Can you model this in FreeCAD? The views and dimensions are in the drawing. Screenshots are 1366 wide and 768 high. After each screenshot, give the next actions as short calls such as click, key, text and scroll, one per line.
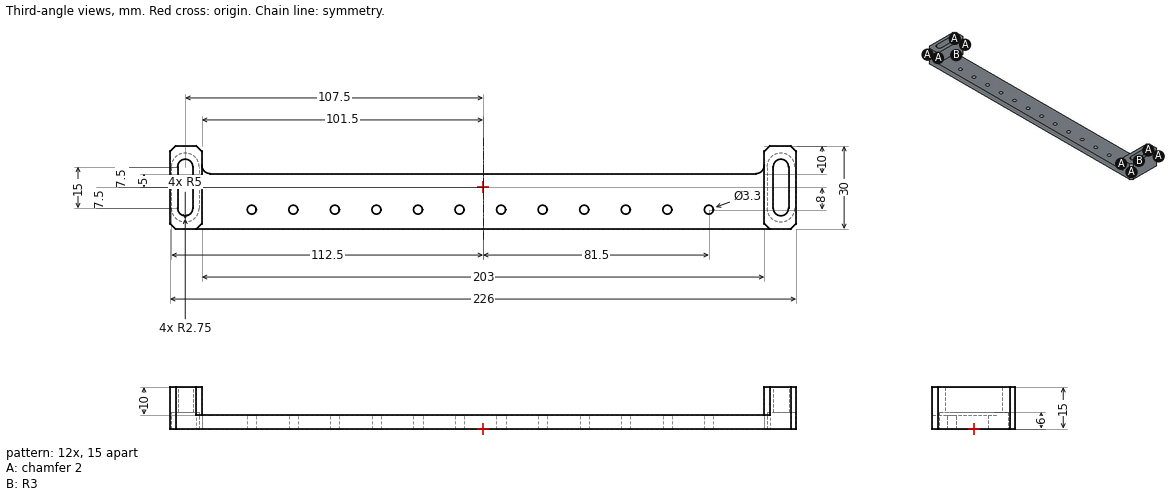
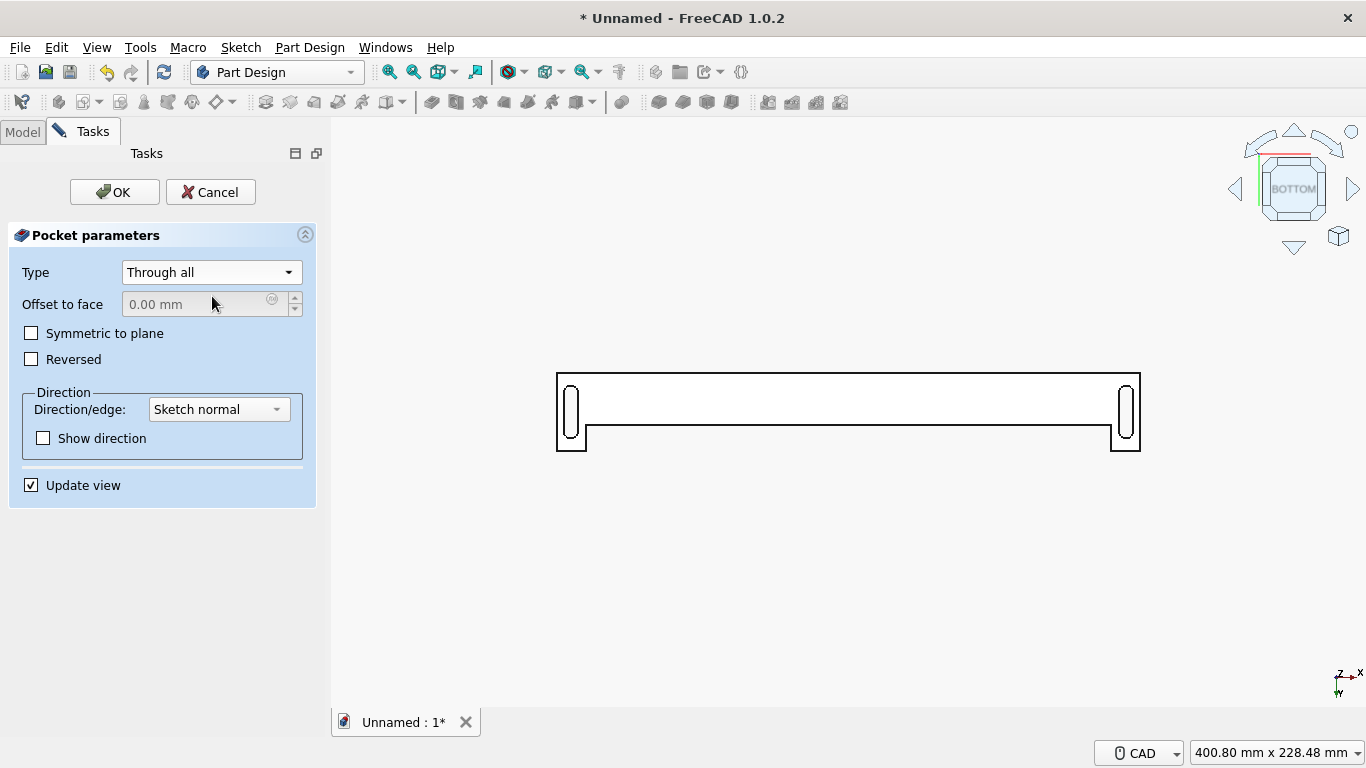
click(115, 192)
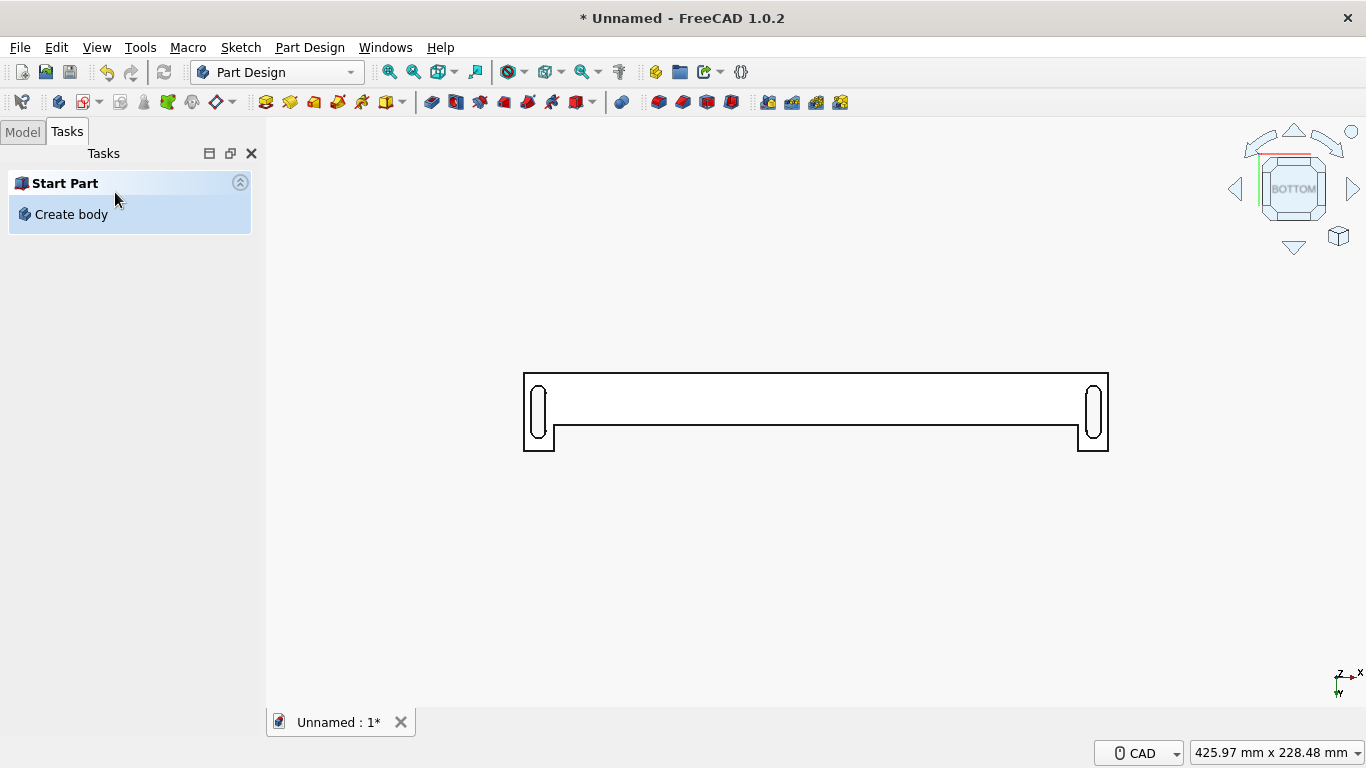
click(84, 102)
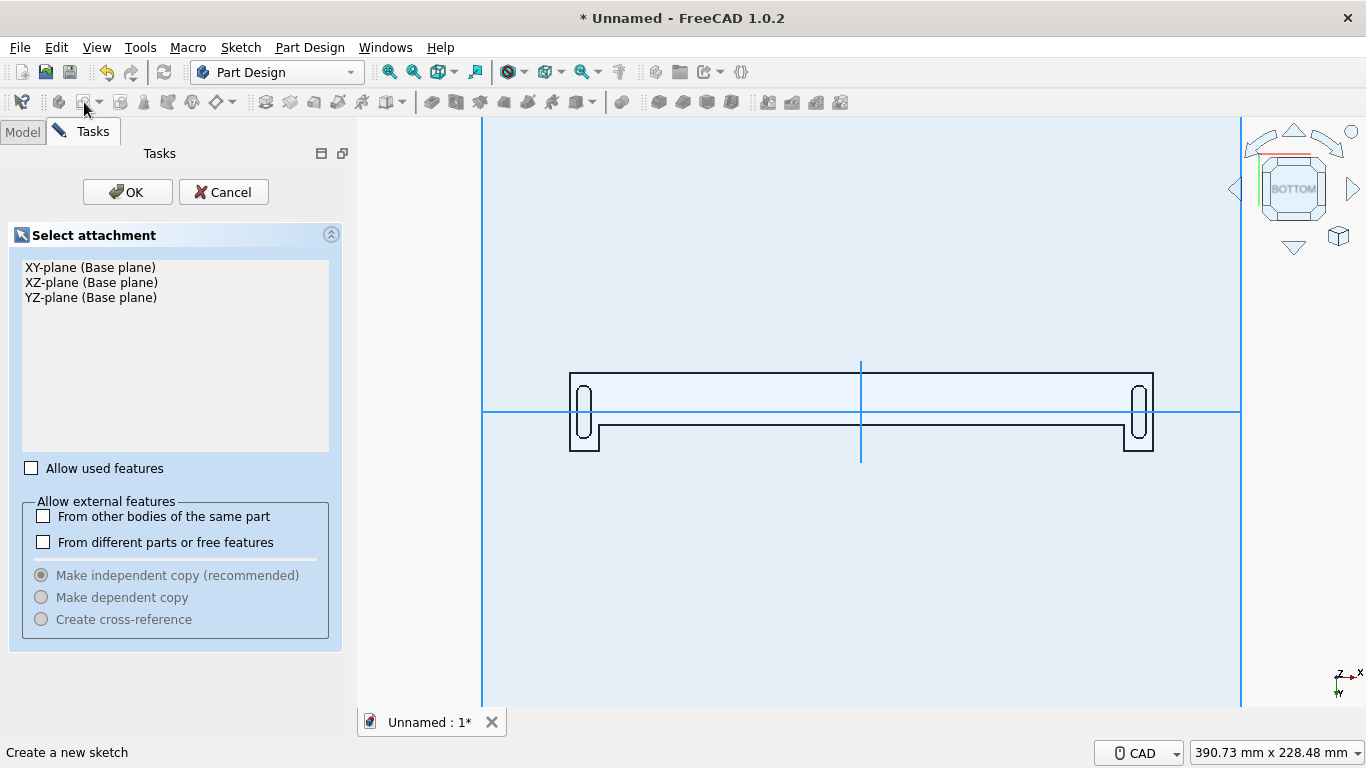
click(82, 268)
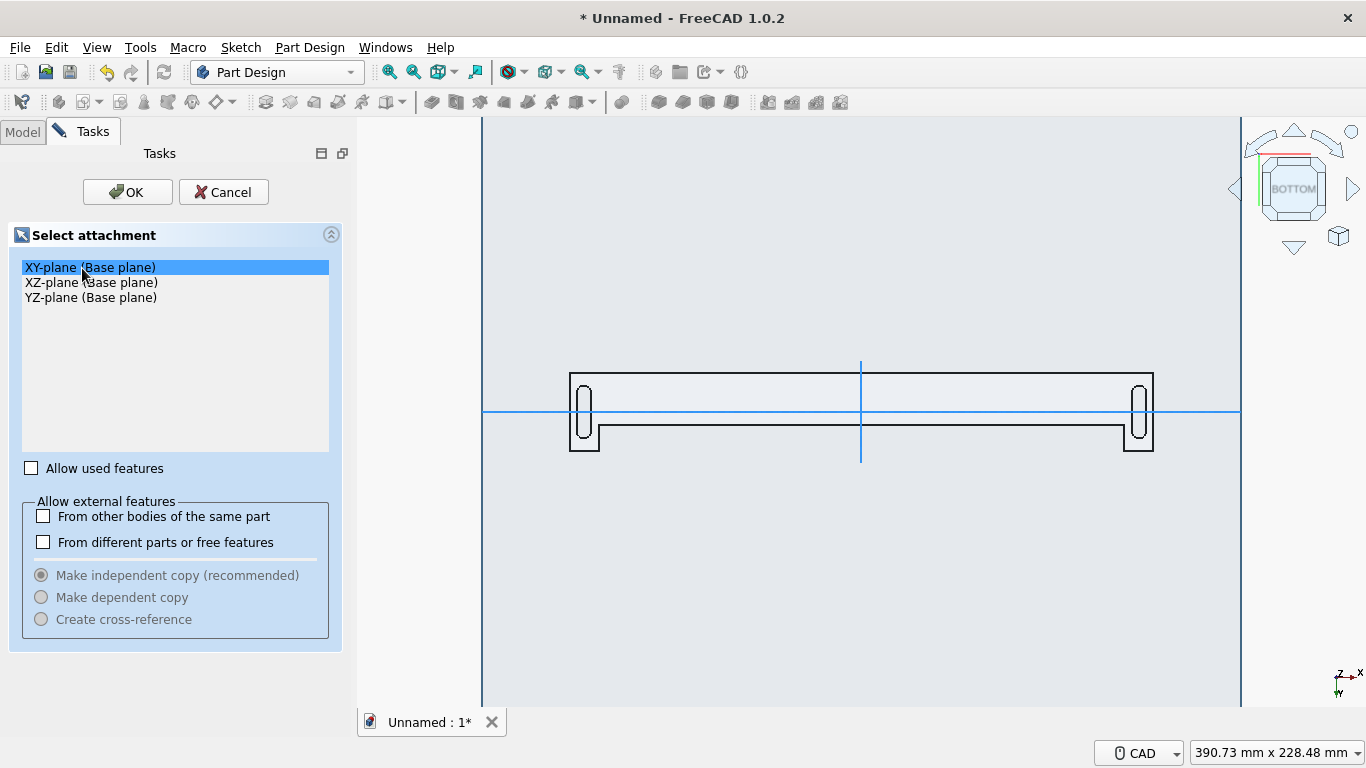
click(128, 192)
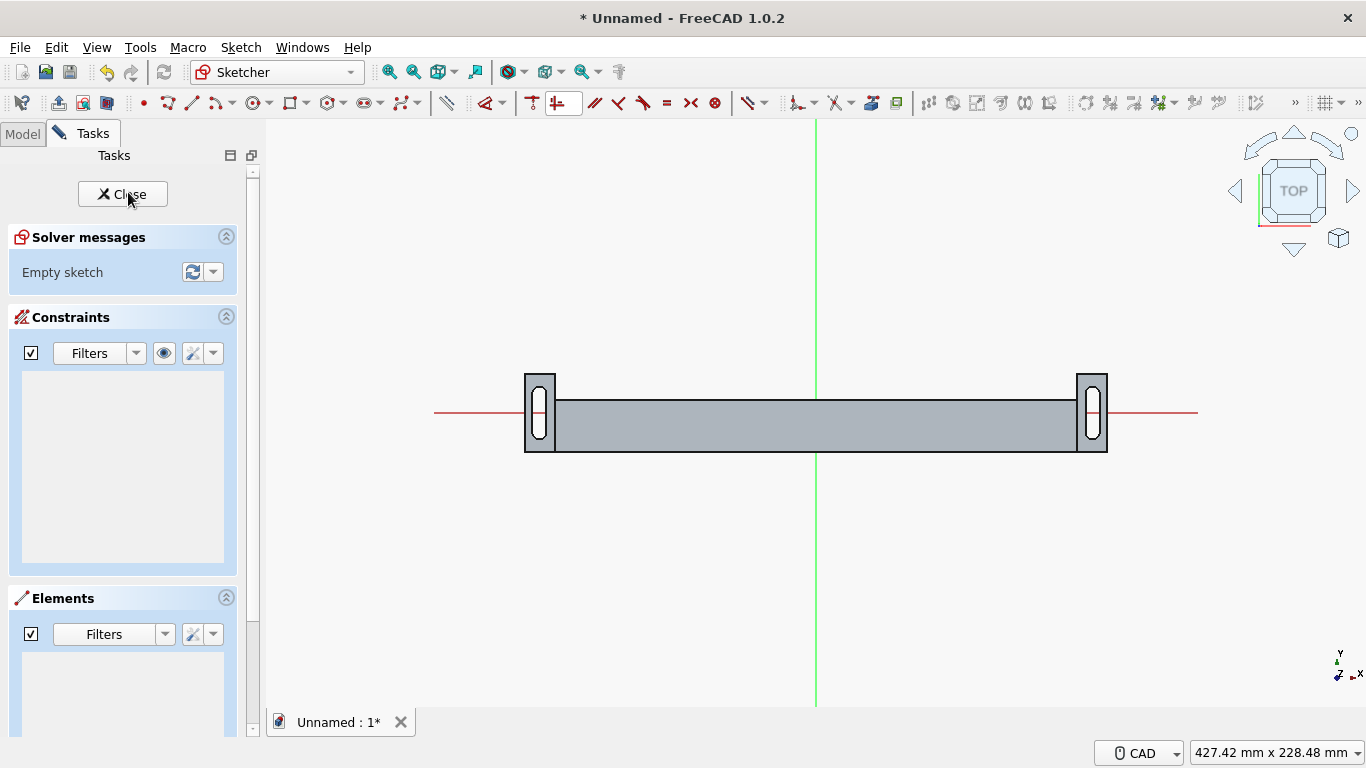
key(q)
key(s)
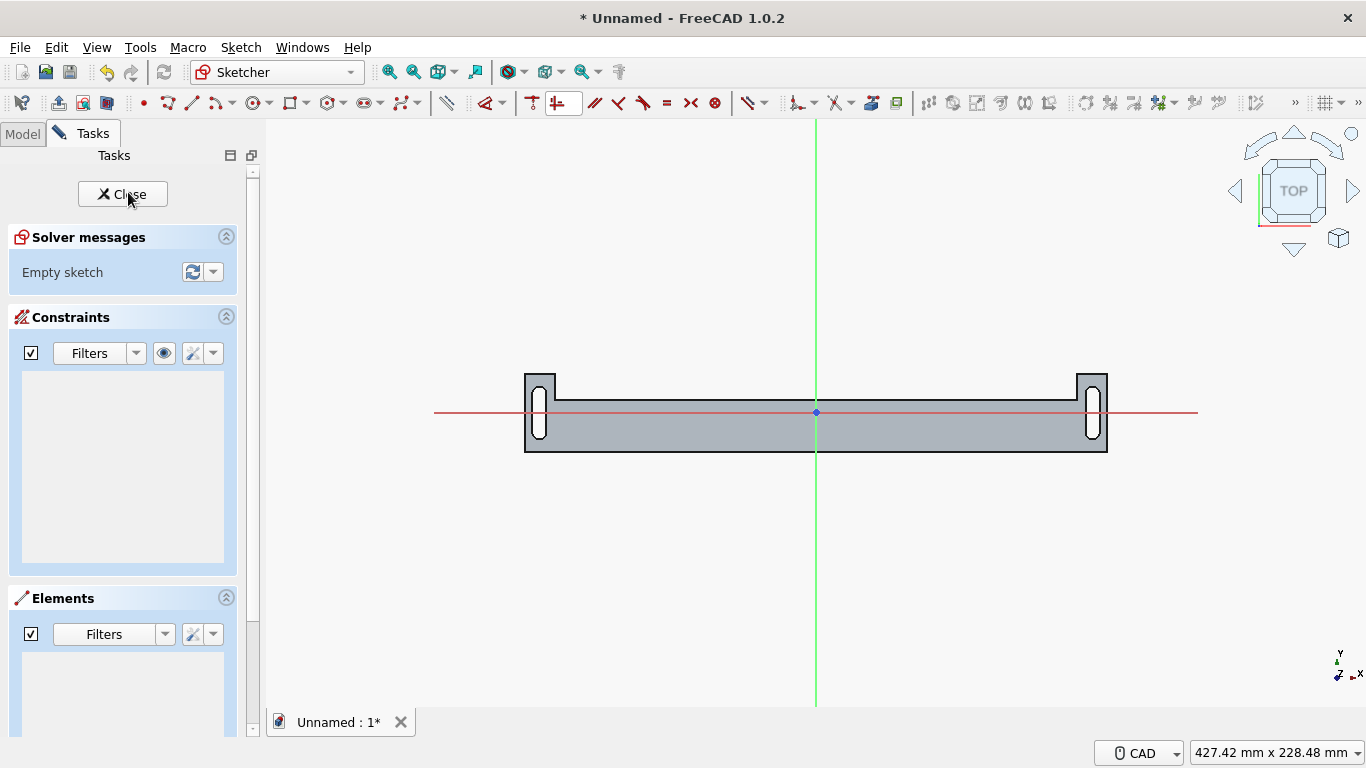
key(g)
key(s)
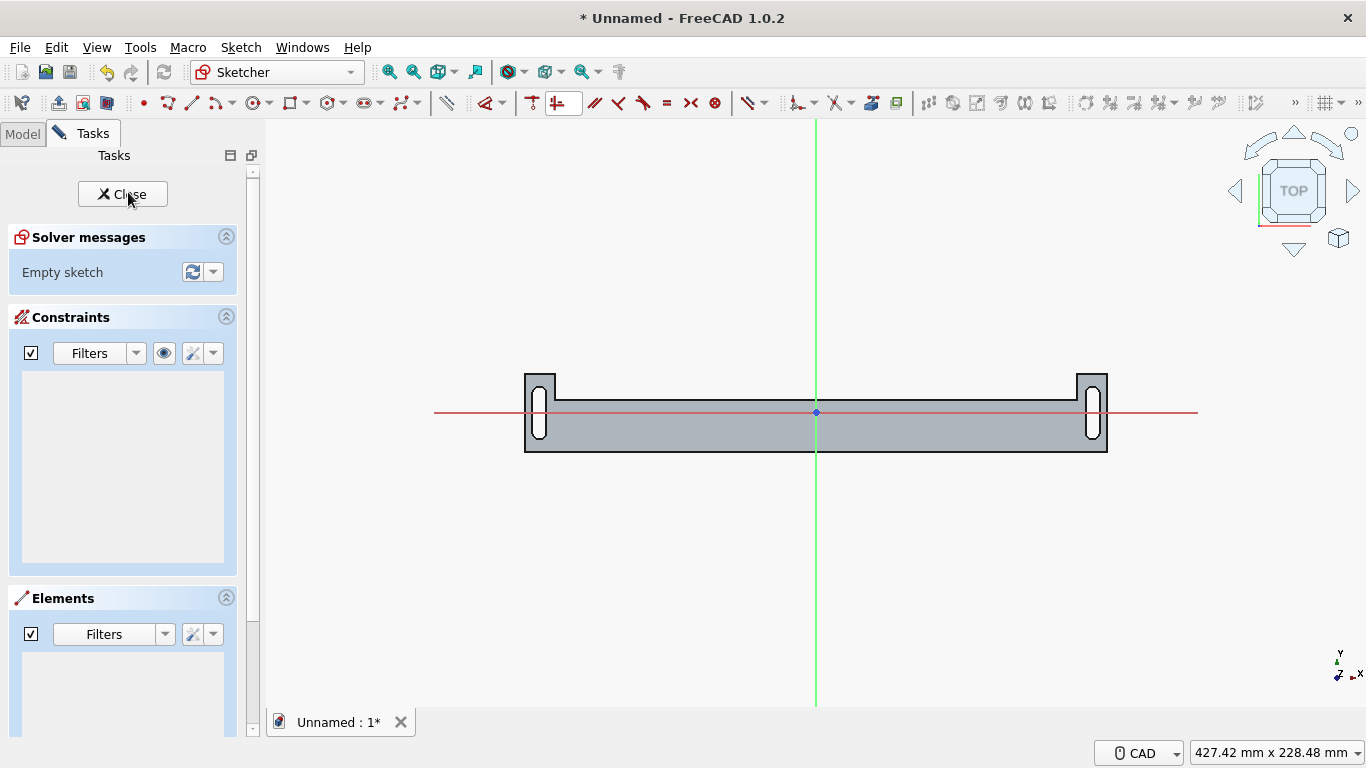
scroll(539, 432, up, 3)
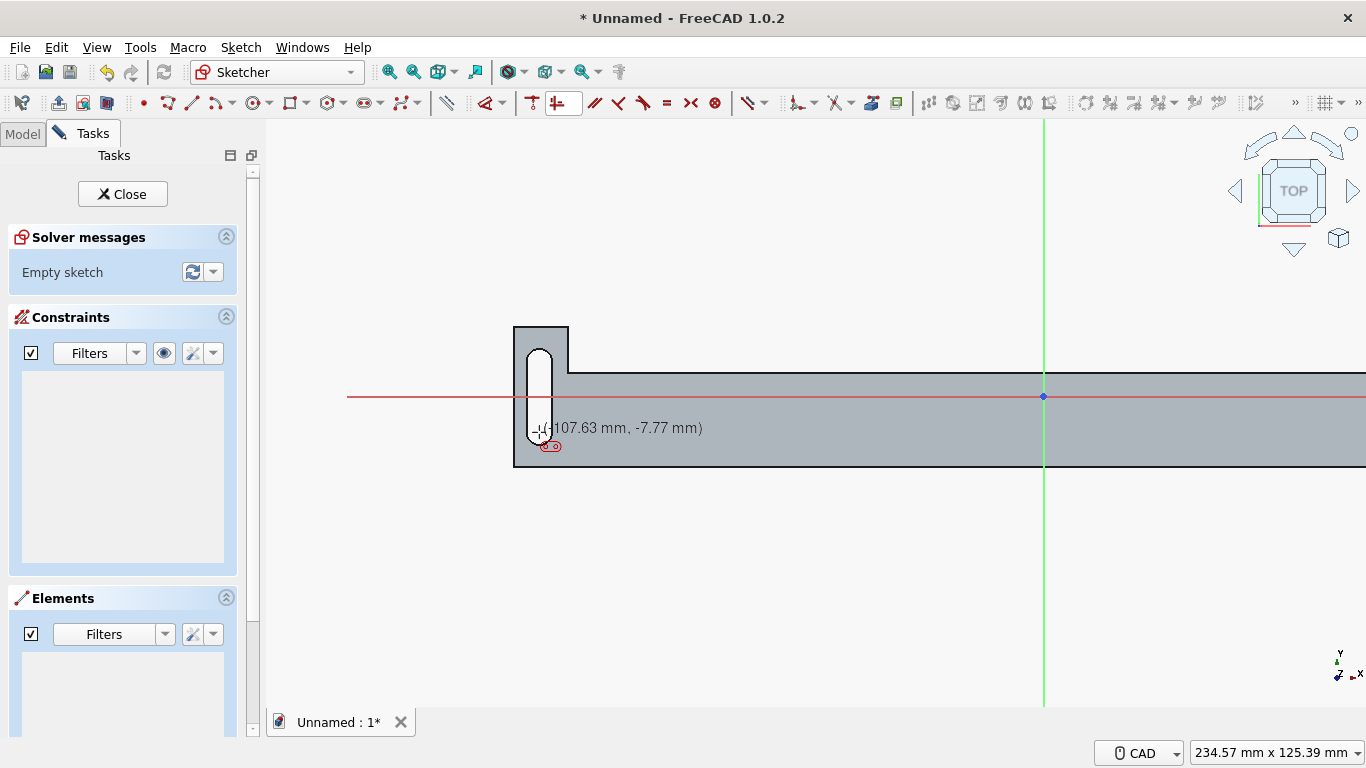
click(539, 432)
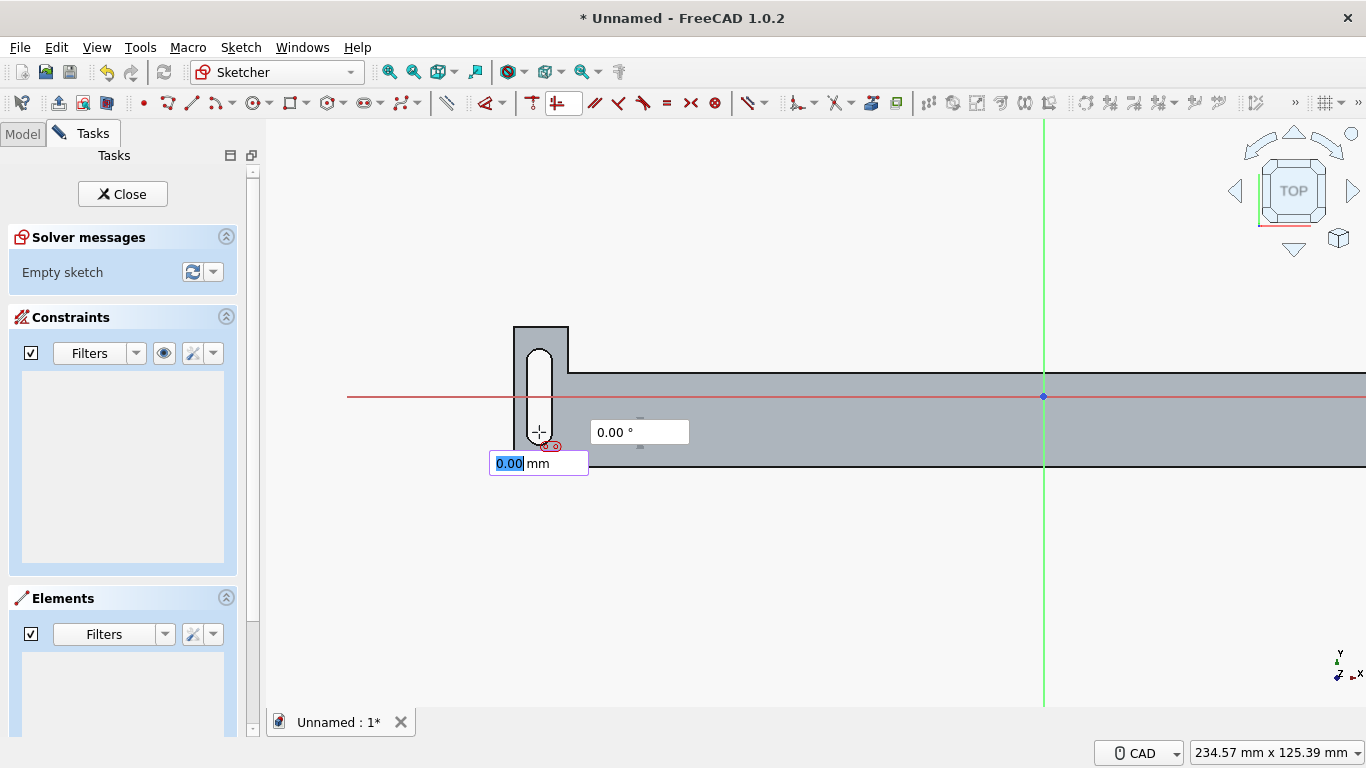
click(539, 362)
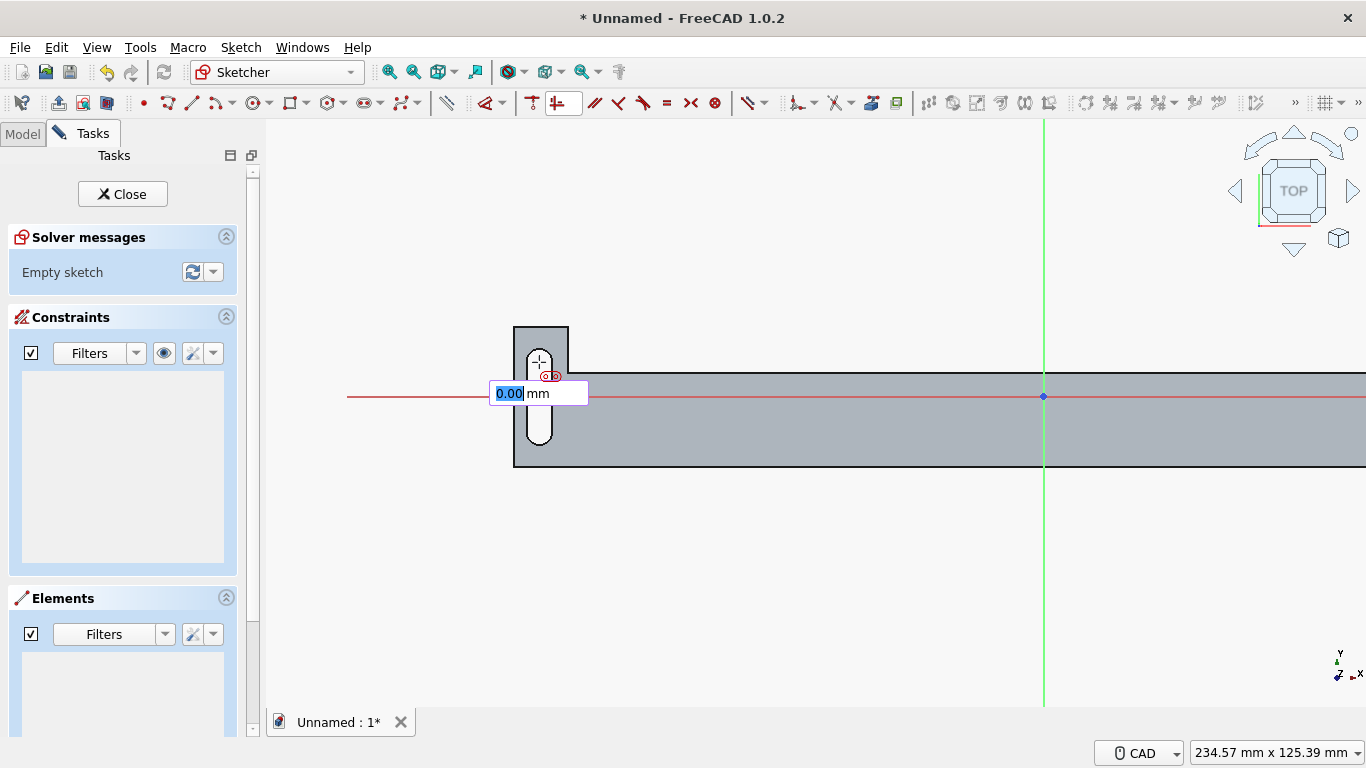
scroll(563, 386, up, 3)